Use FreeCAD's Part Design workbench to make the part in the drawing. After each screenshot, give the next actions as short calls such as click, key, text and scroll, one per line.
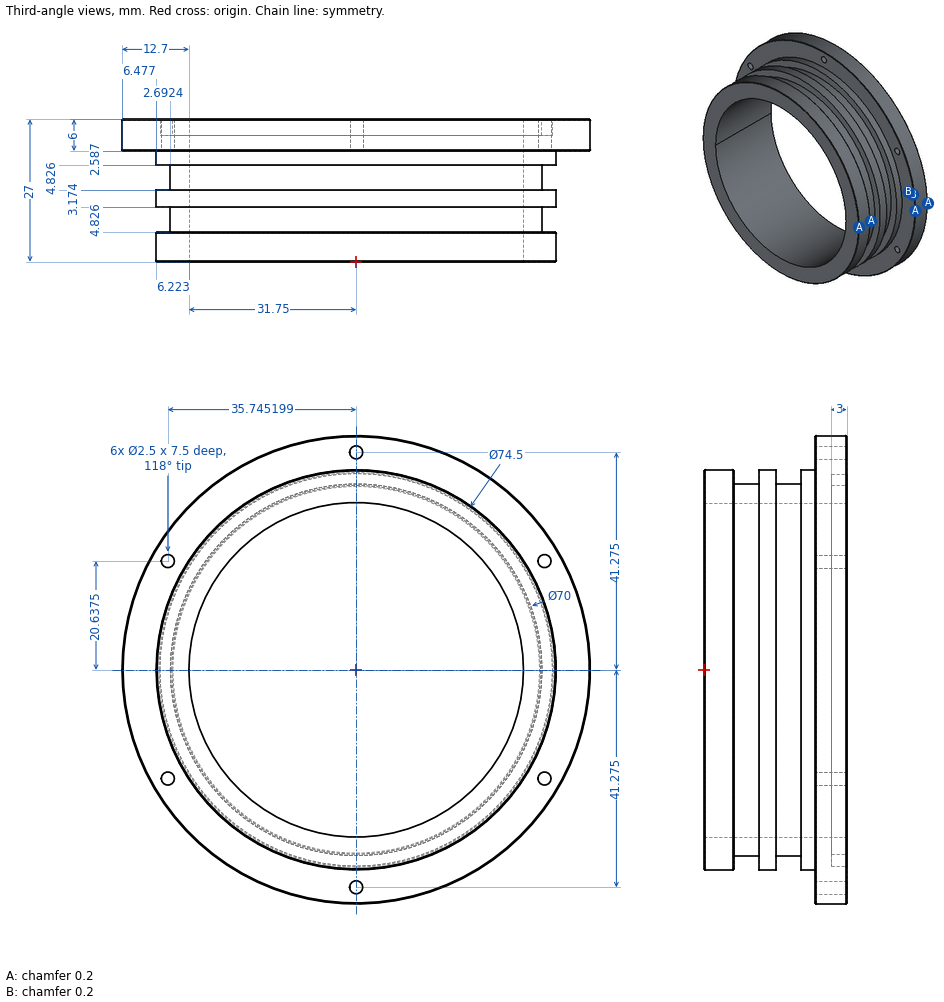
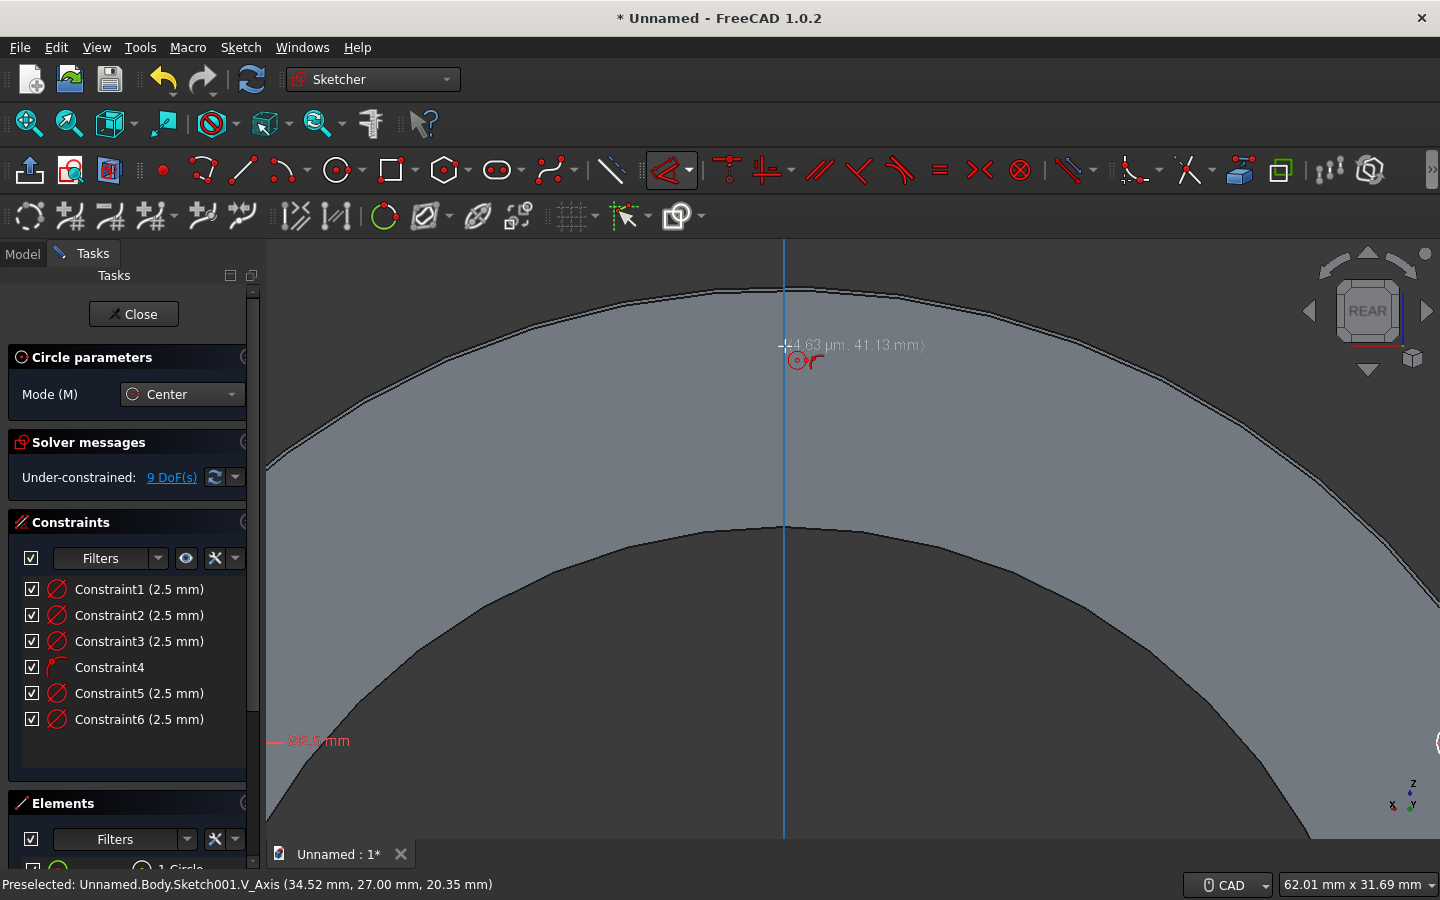
scroll(785, 346, down, 7)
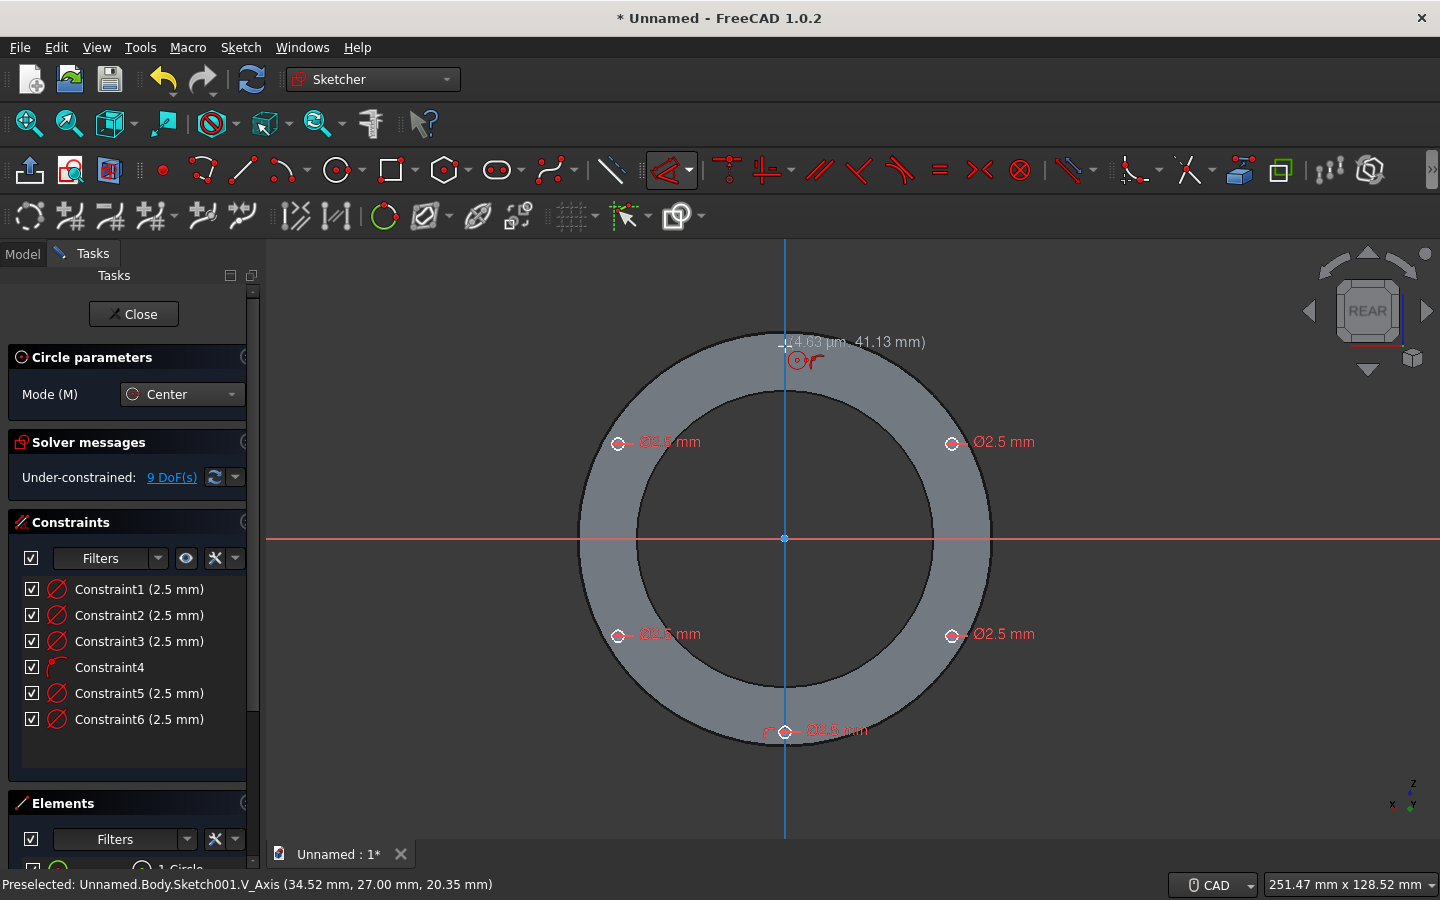
click(785, 346)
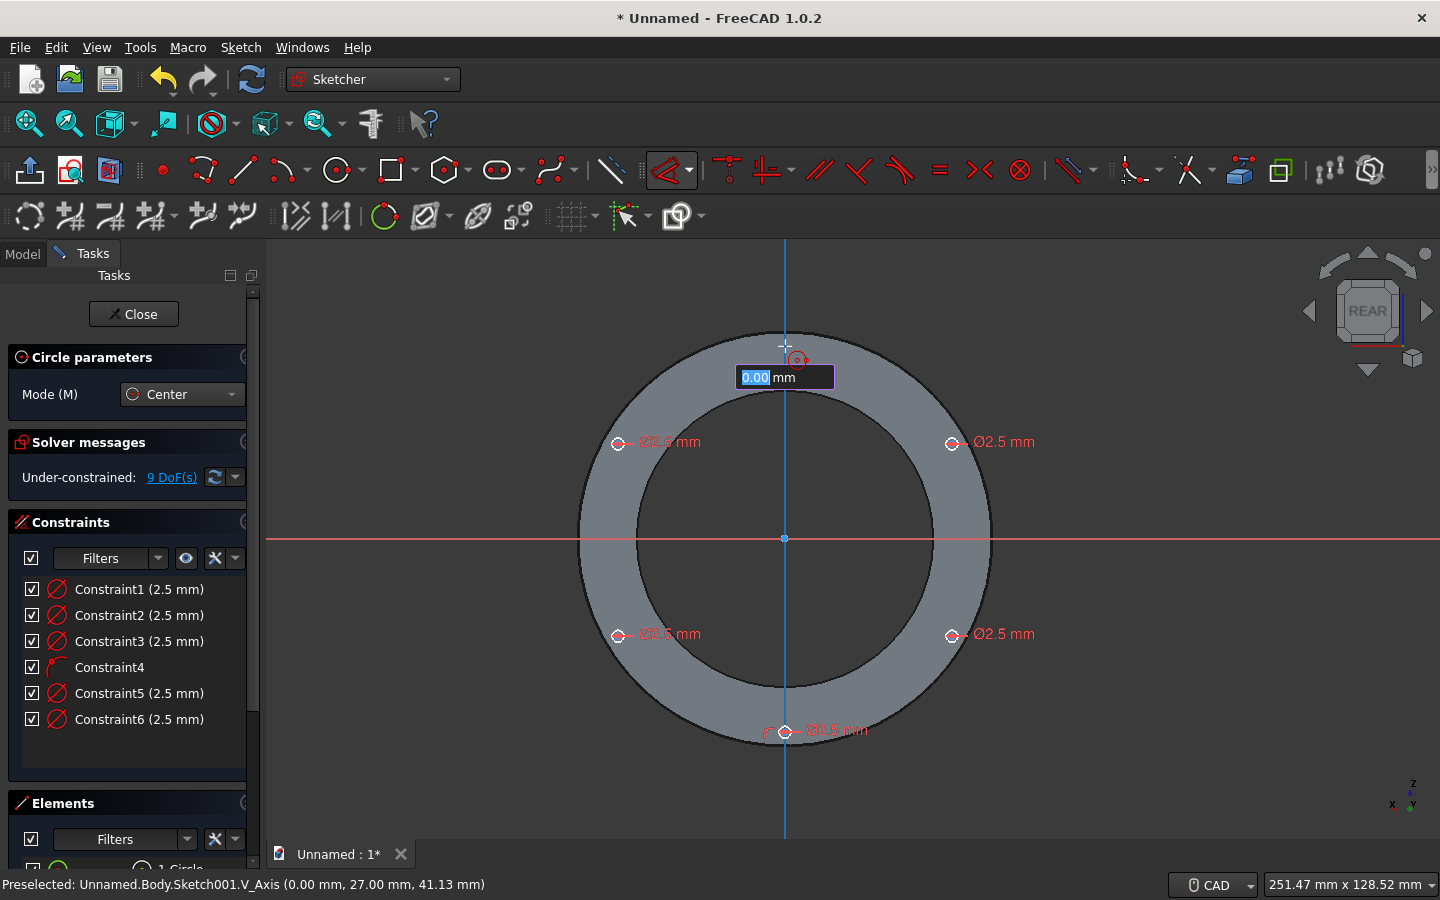
scroll(790, 344, up, 6)
move(790, 345)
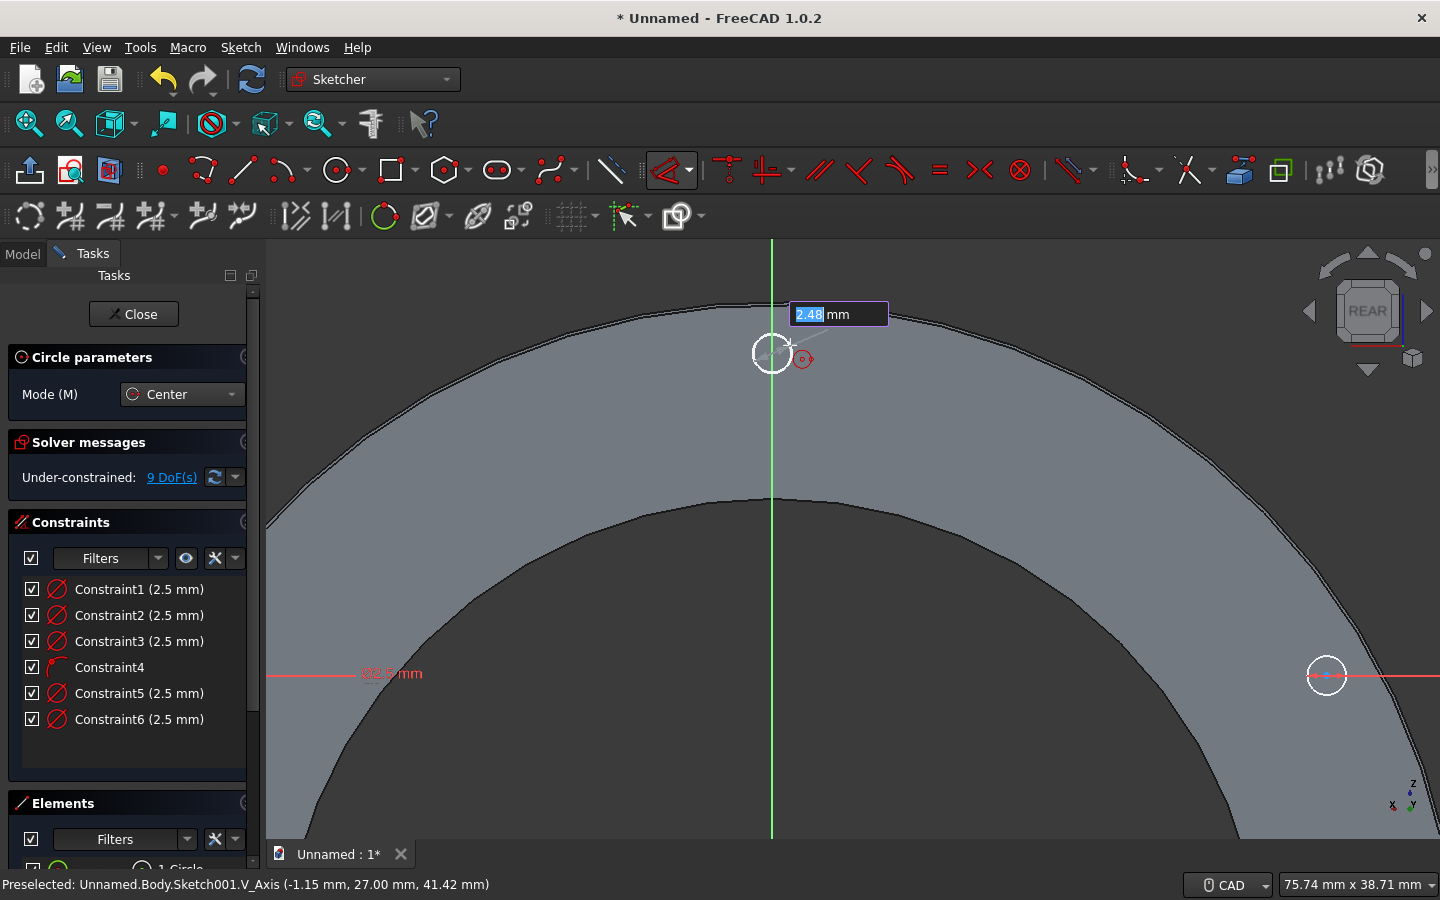
text(2.5)
key(Return)
key(Escape)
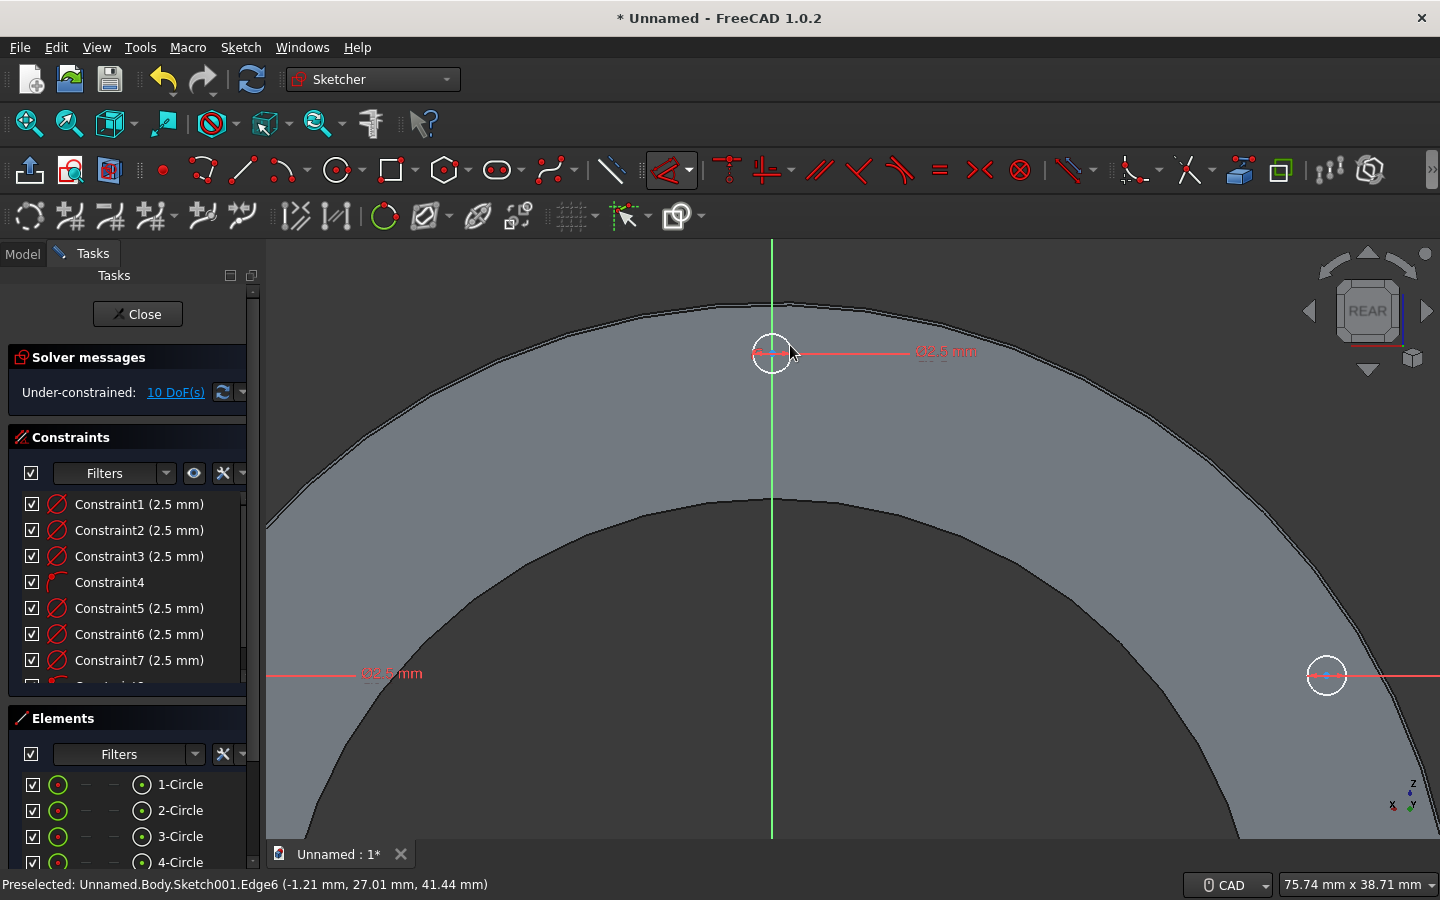
scroll(790, 344, down, 6)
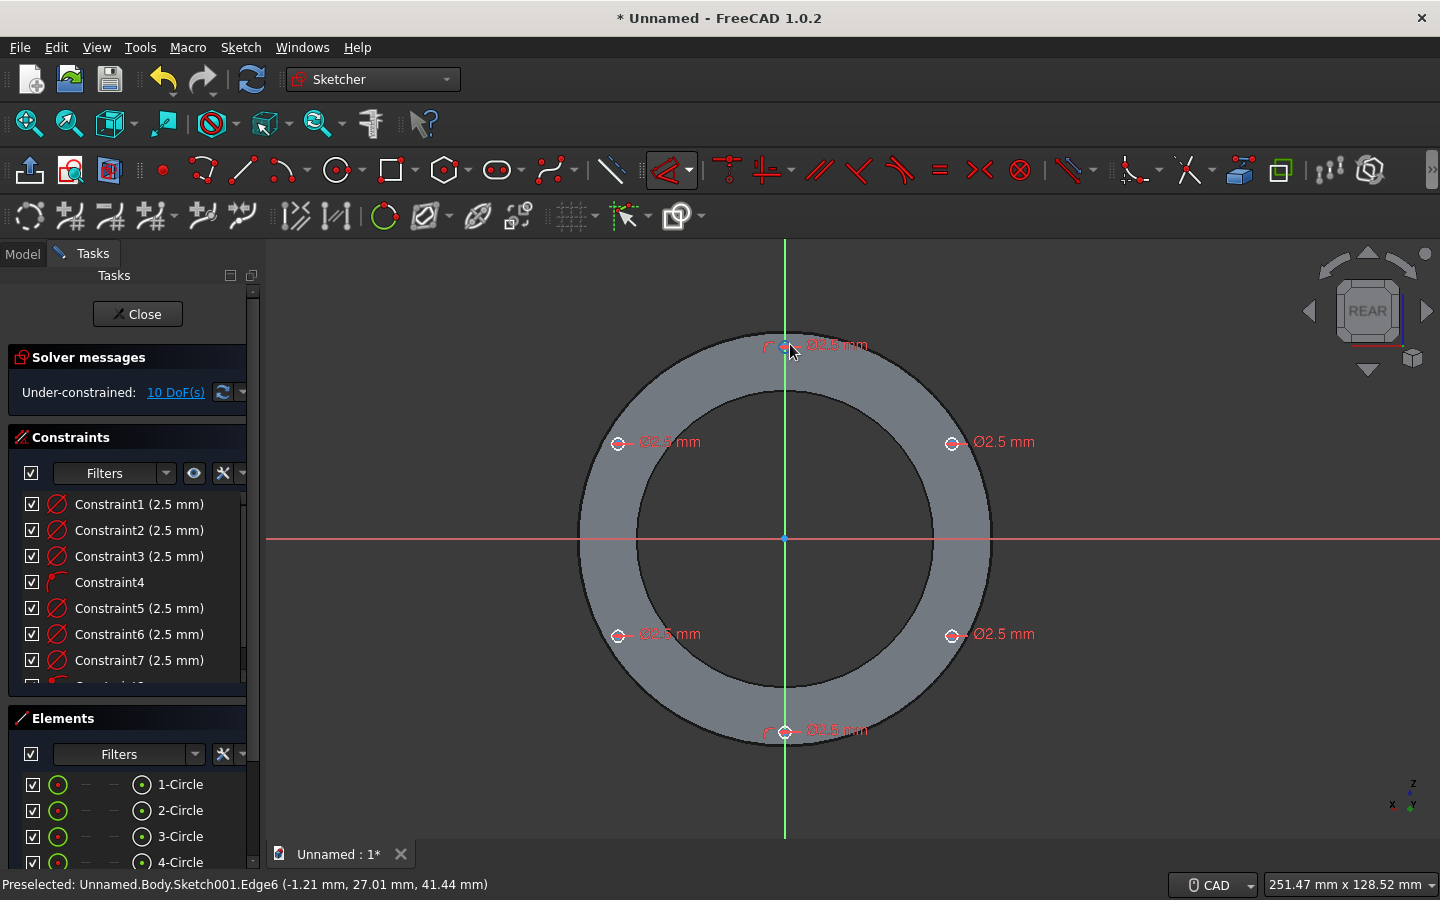
click(952, 444)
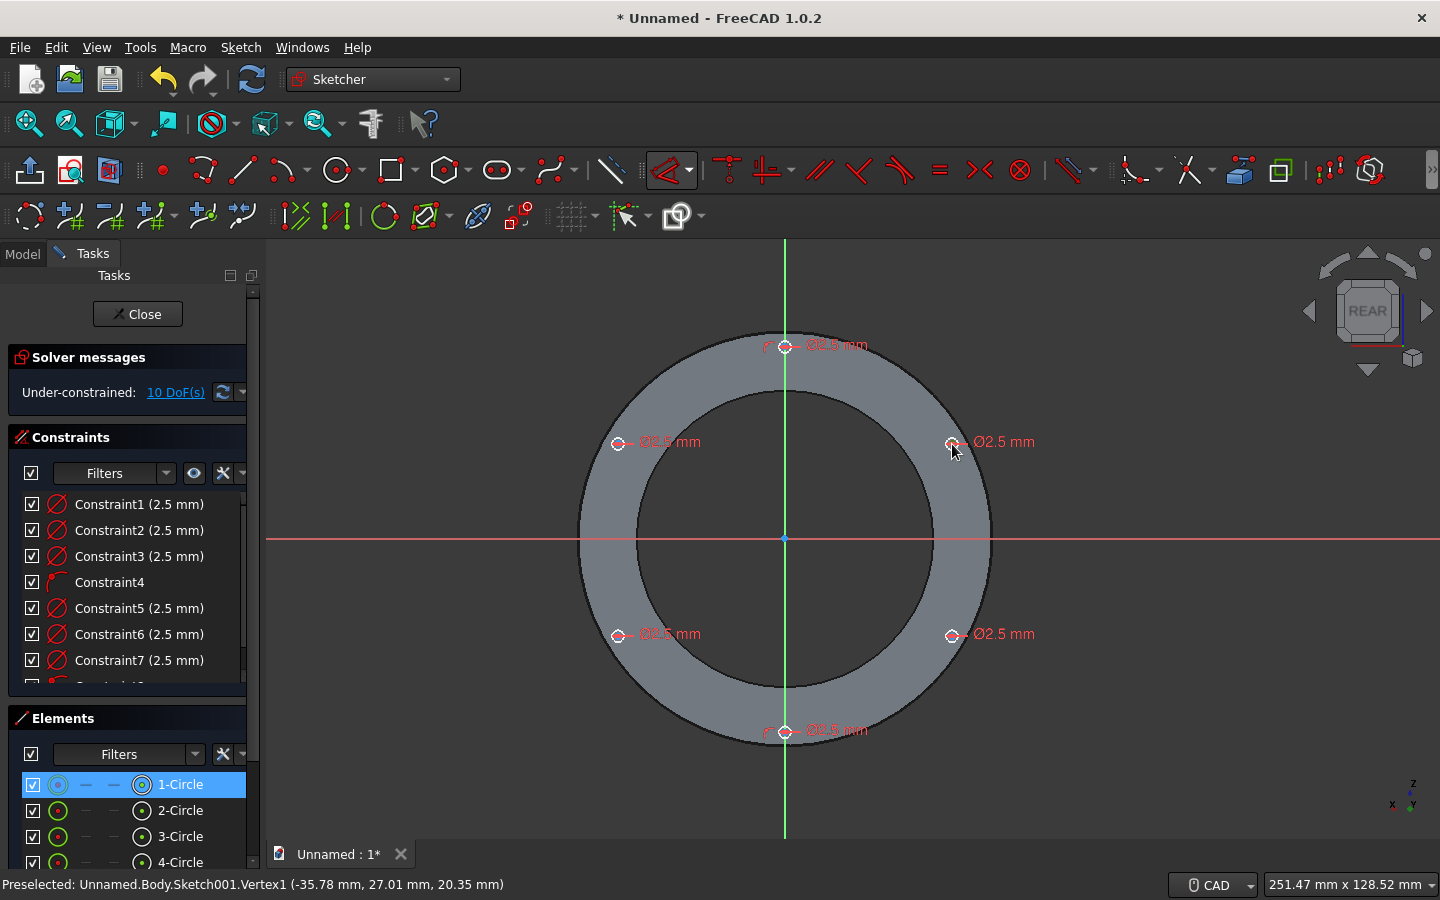
click(952, 636)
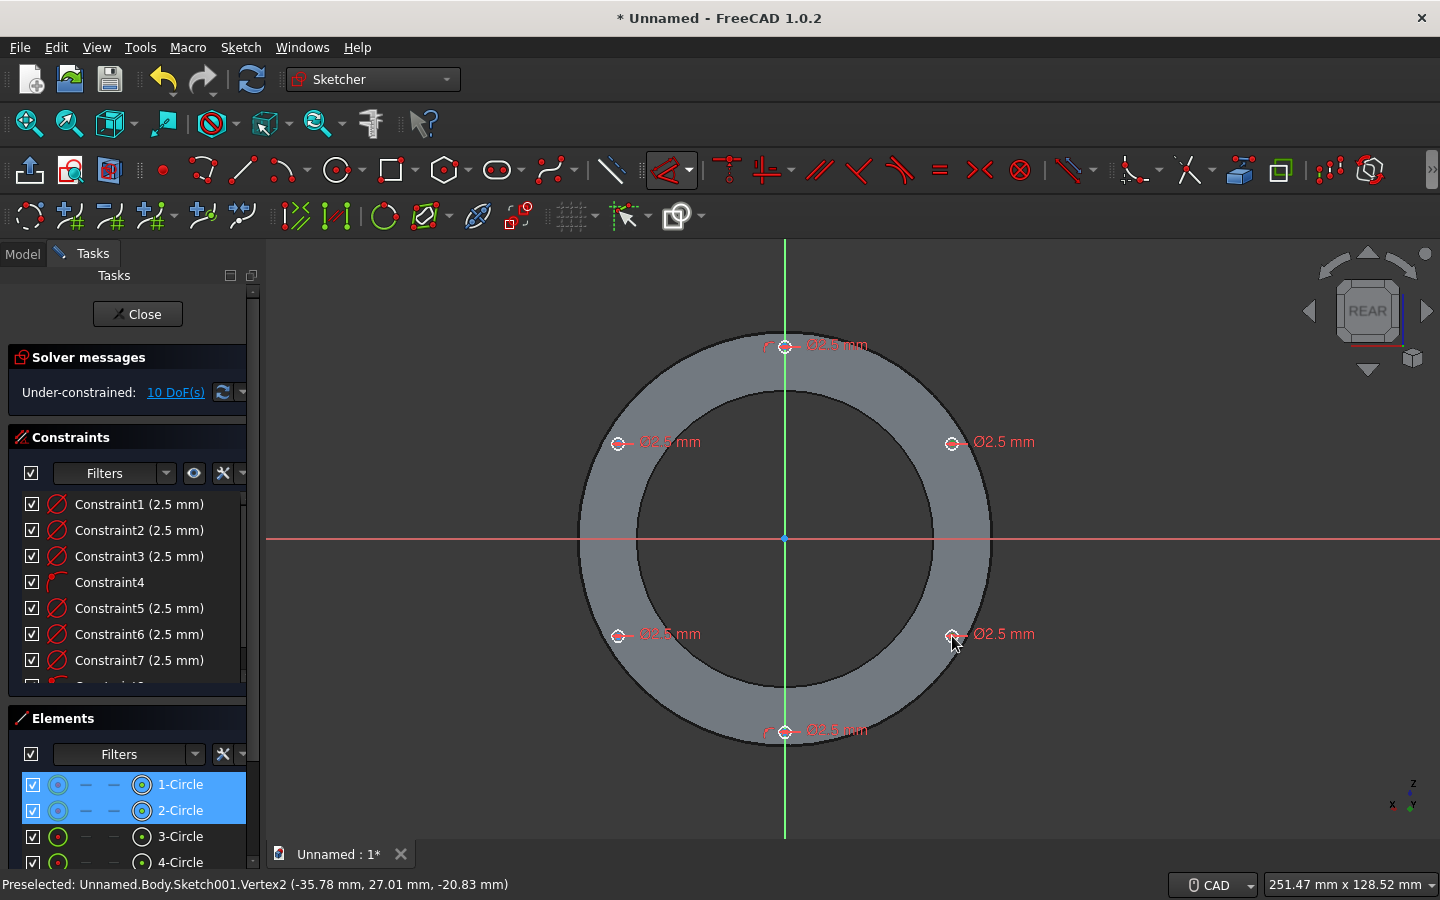
click(364, 539)